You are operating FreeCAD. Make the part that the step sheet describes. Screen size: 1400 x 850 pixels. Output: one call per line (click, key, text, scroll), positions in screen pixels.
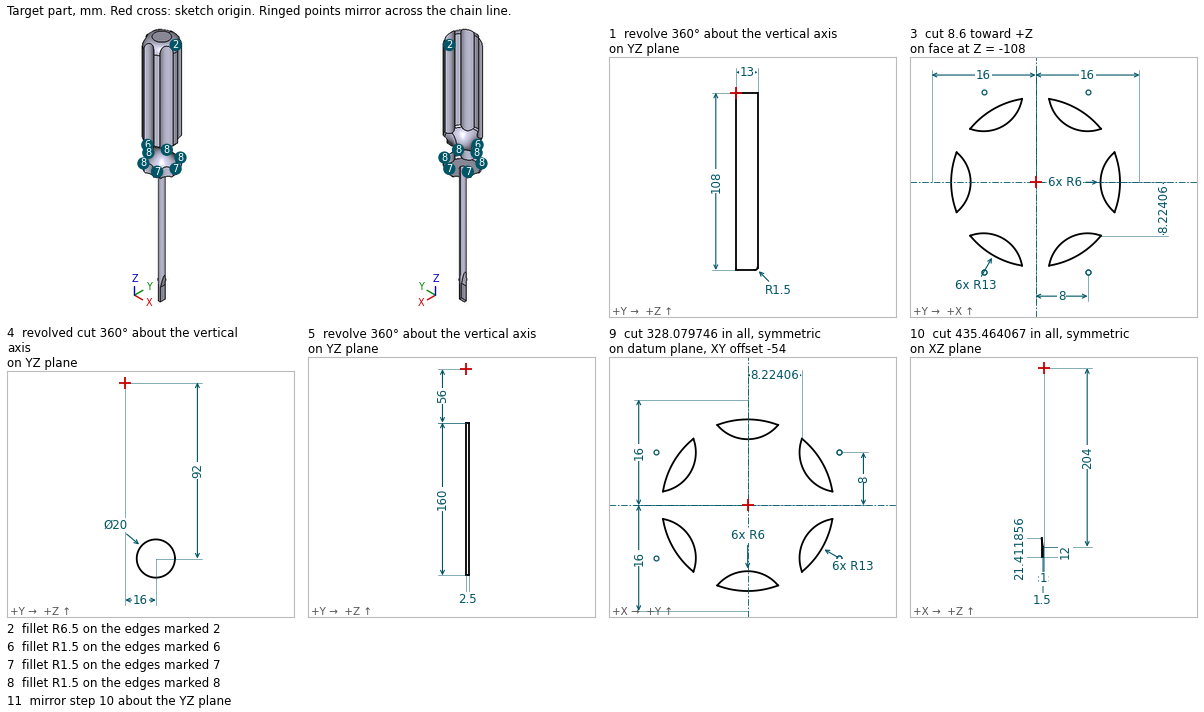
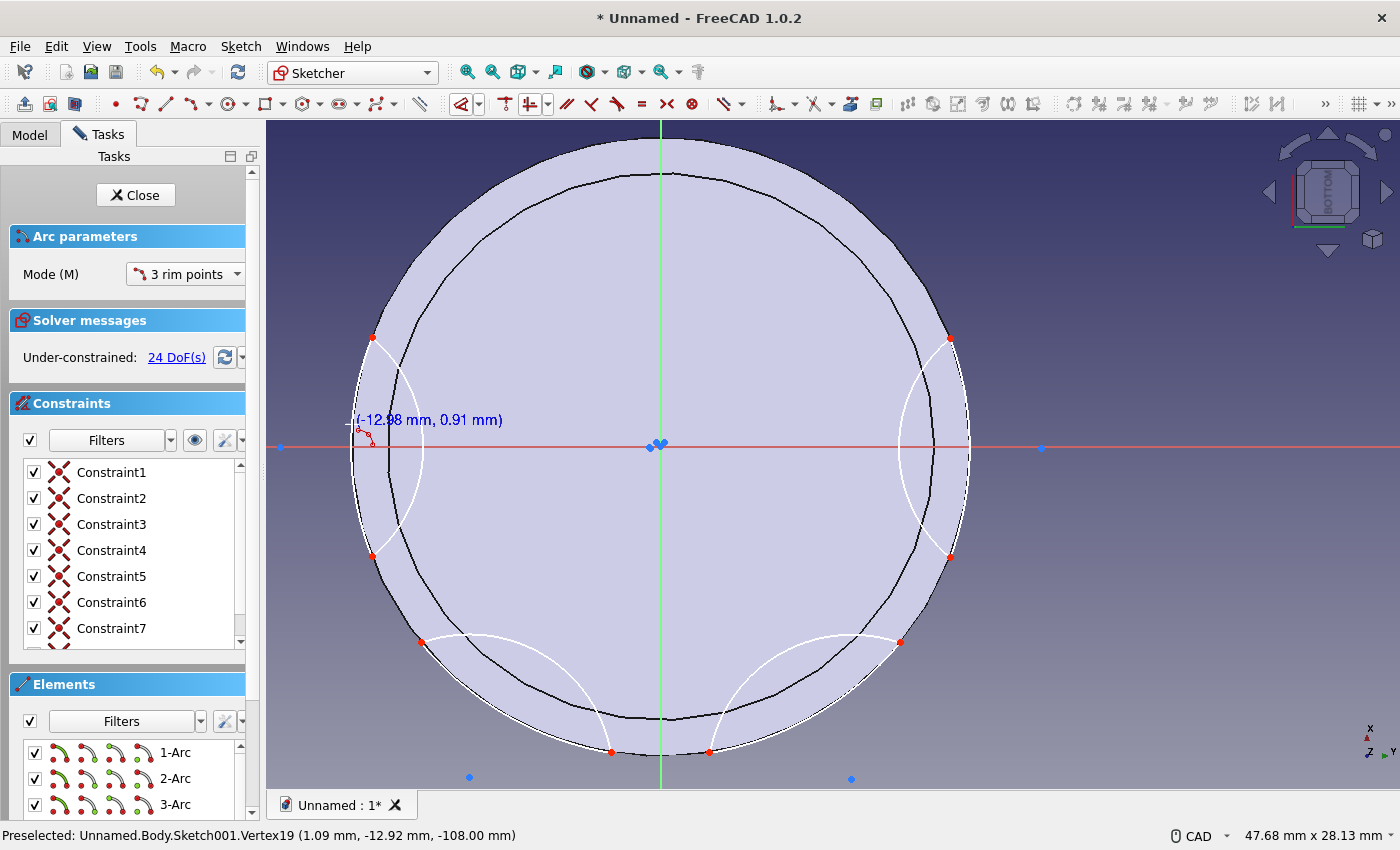
scroll(975, 471, down, 2)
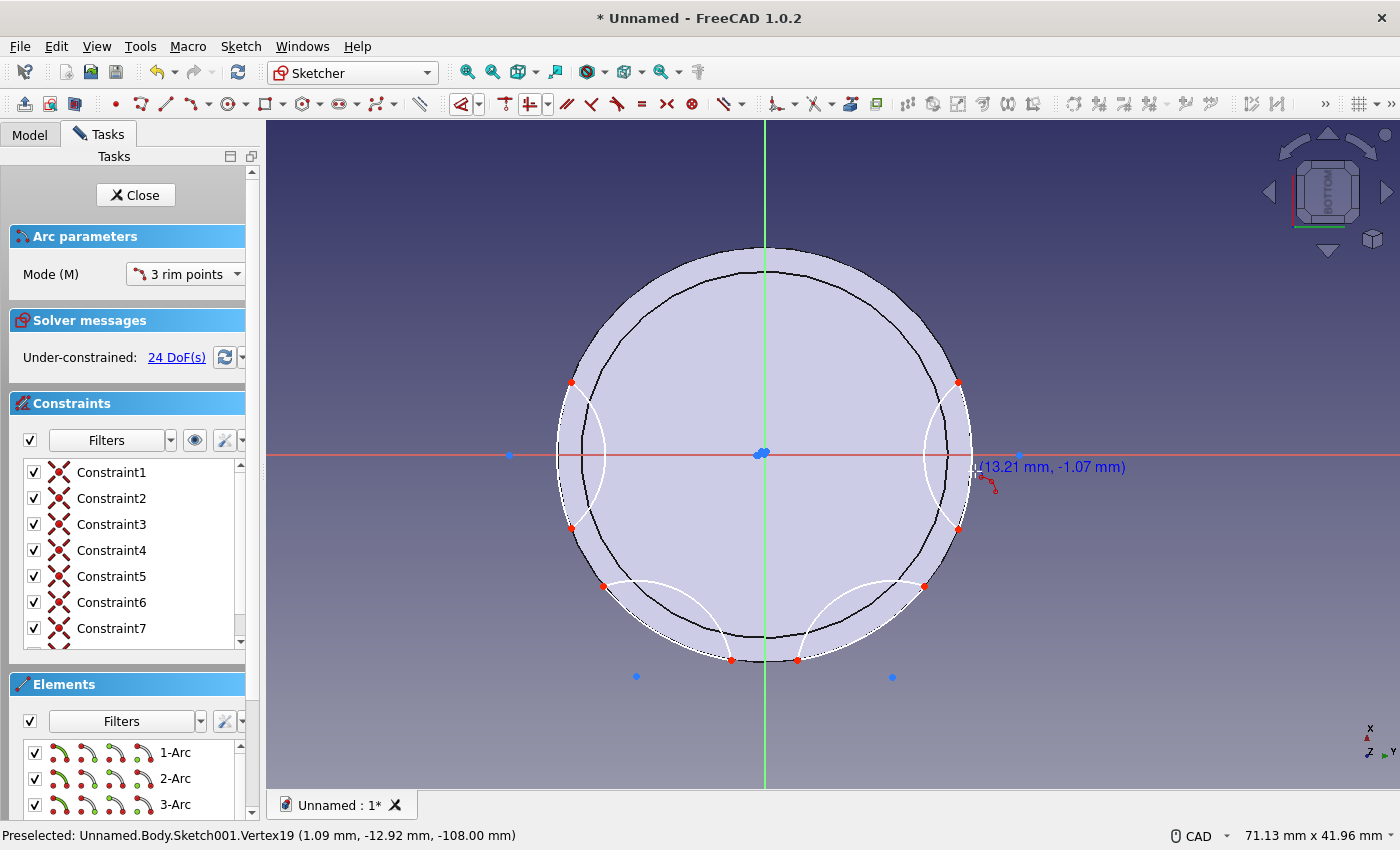
click(731, 250)
click(604, 324)
click(661, 275)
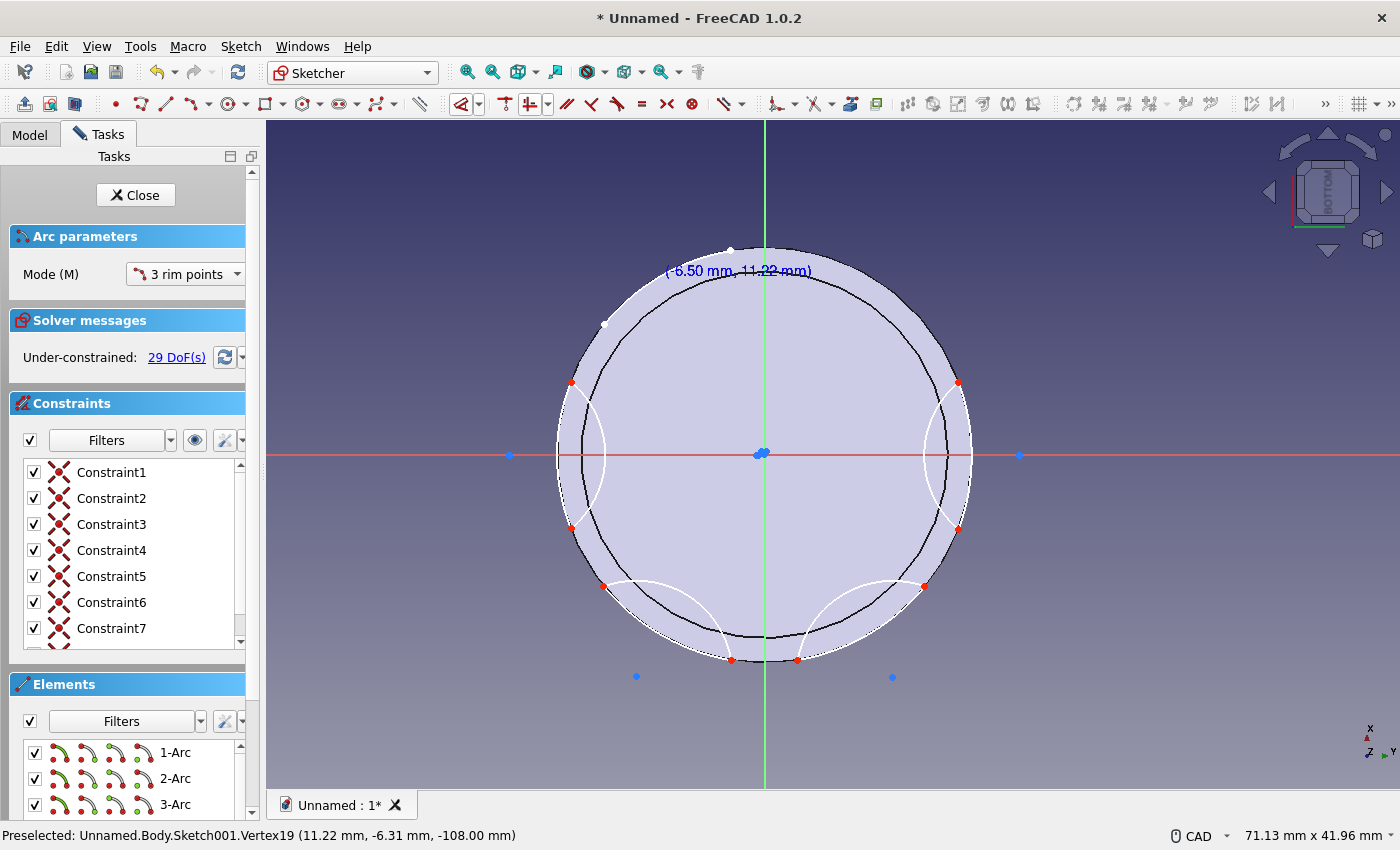
click(604, 325)
click(731, 251)
click(685, 317)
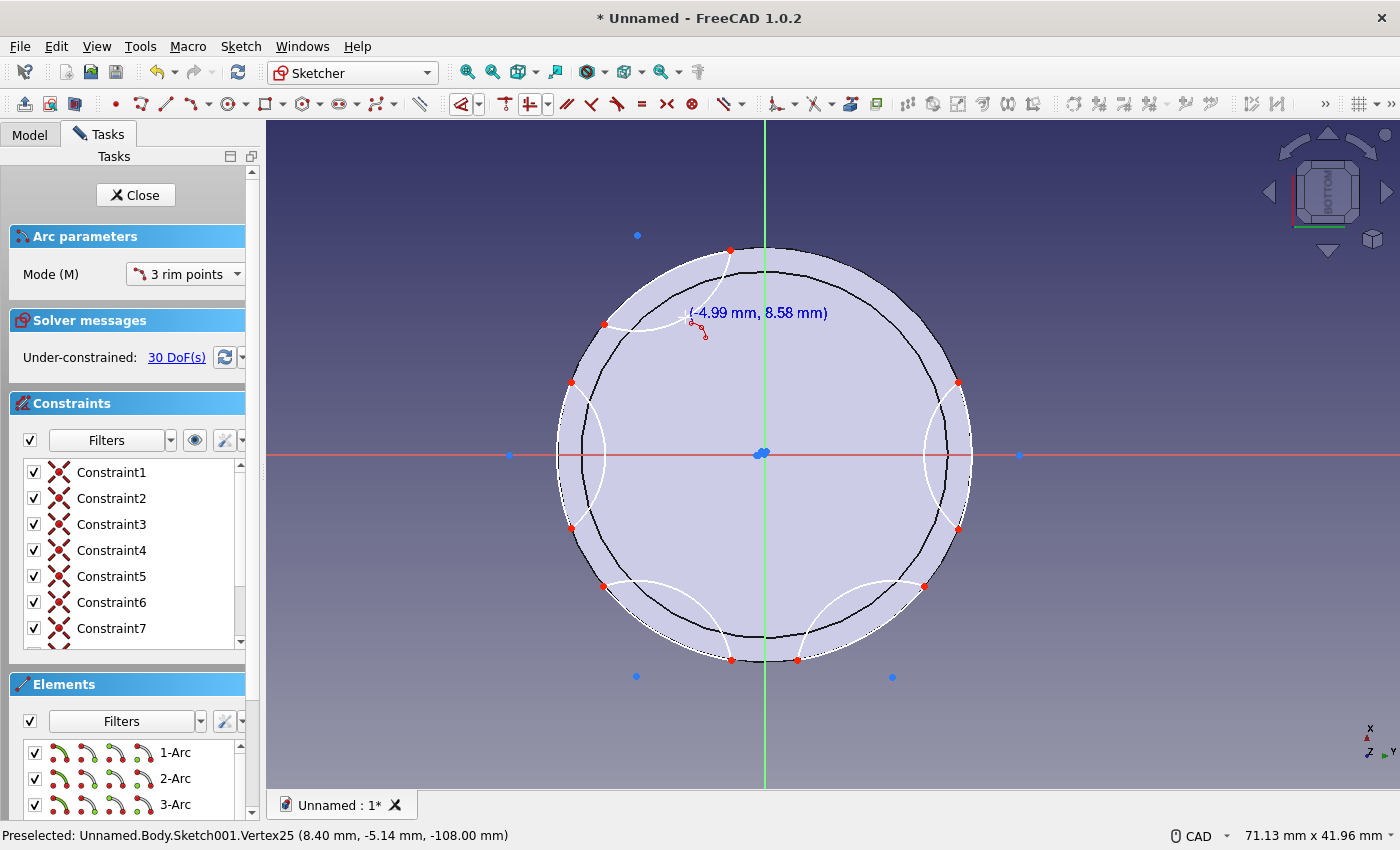
click(798, 250)
click(925, 324)
click(844, 317)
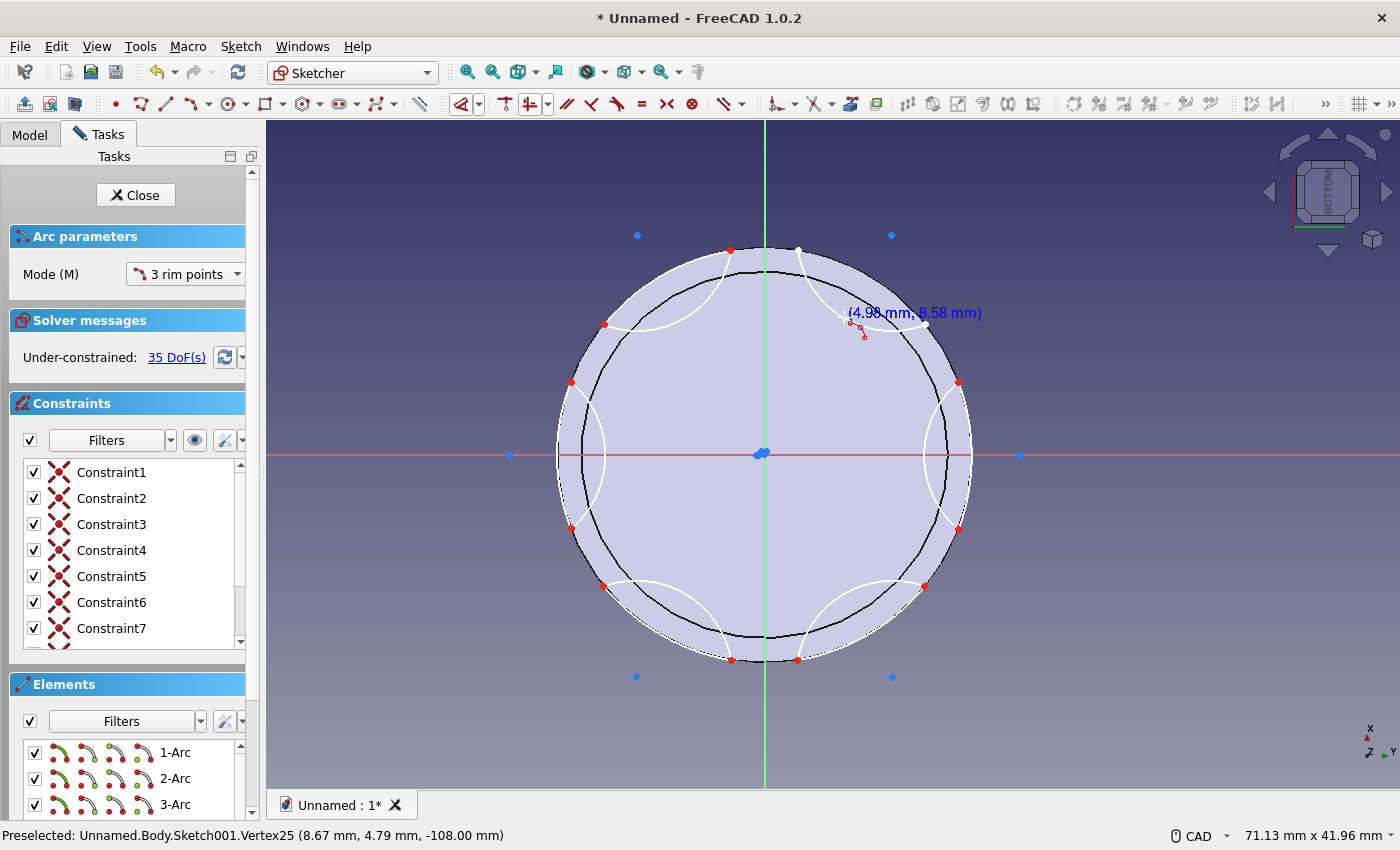
click(925, 325)
click(798, 251)
click(868, 275)
key(Escape)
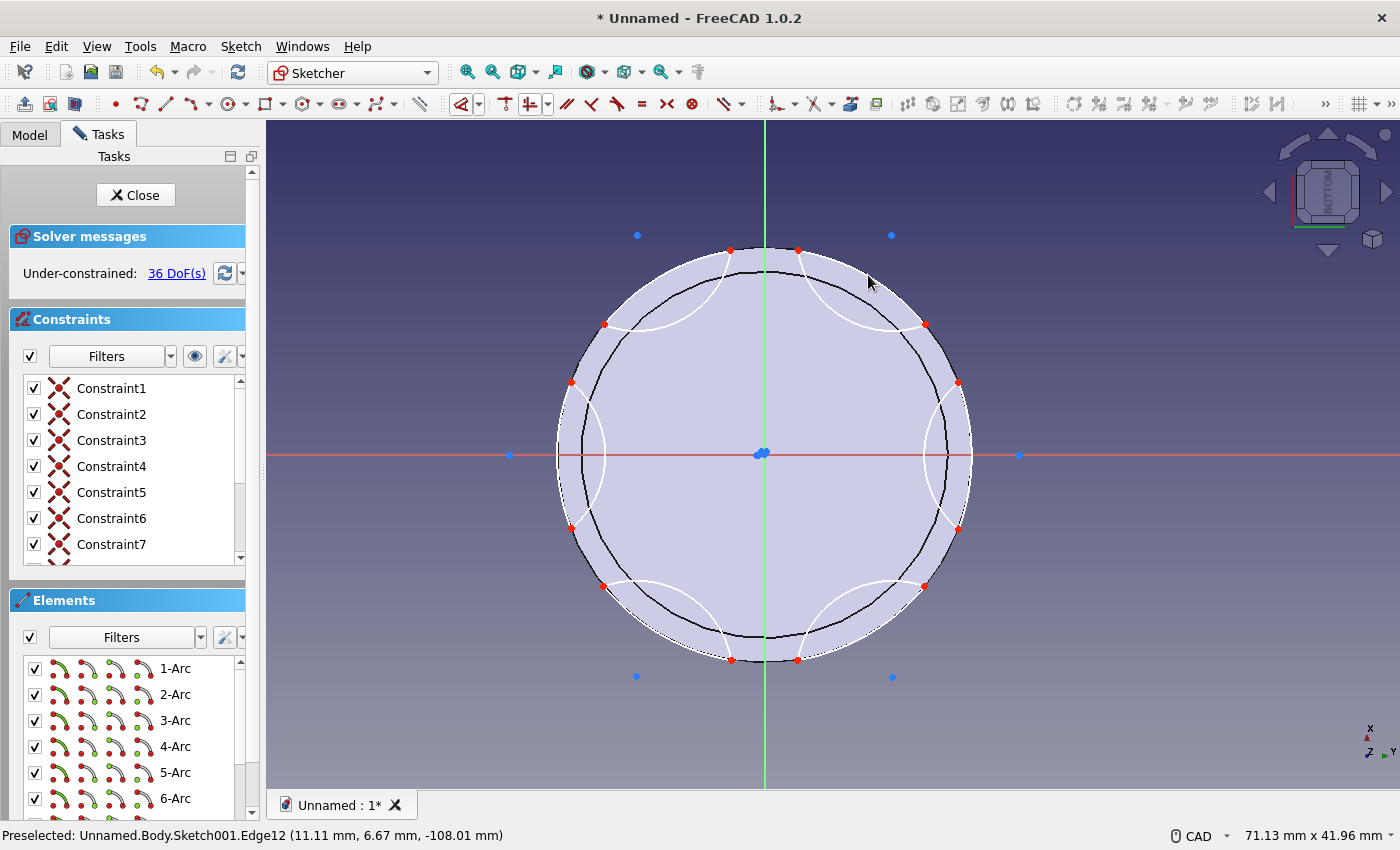
click(970, 486)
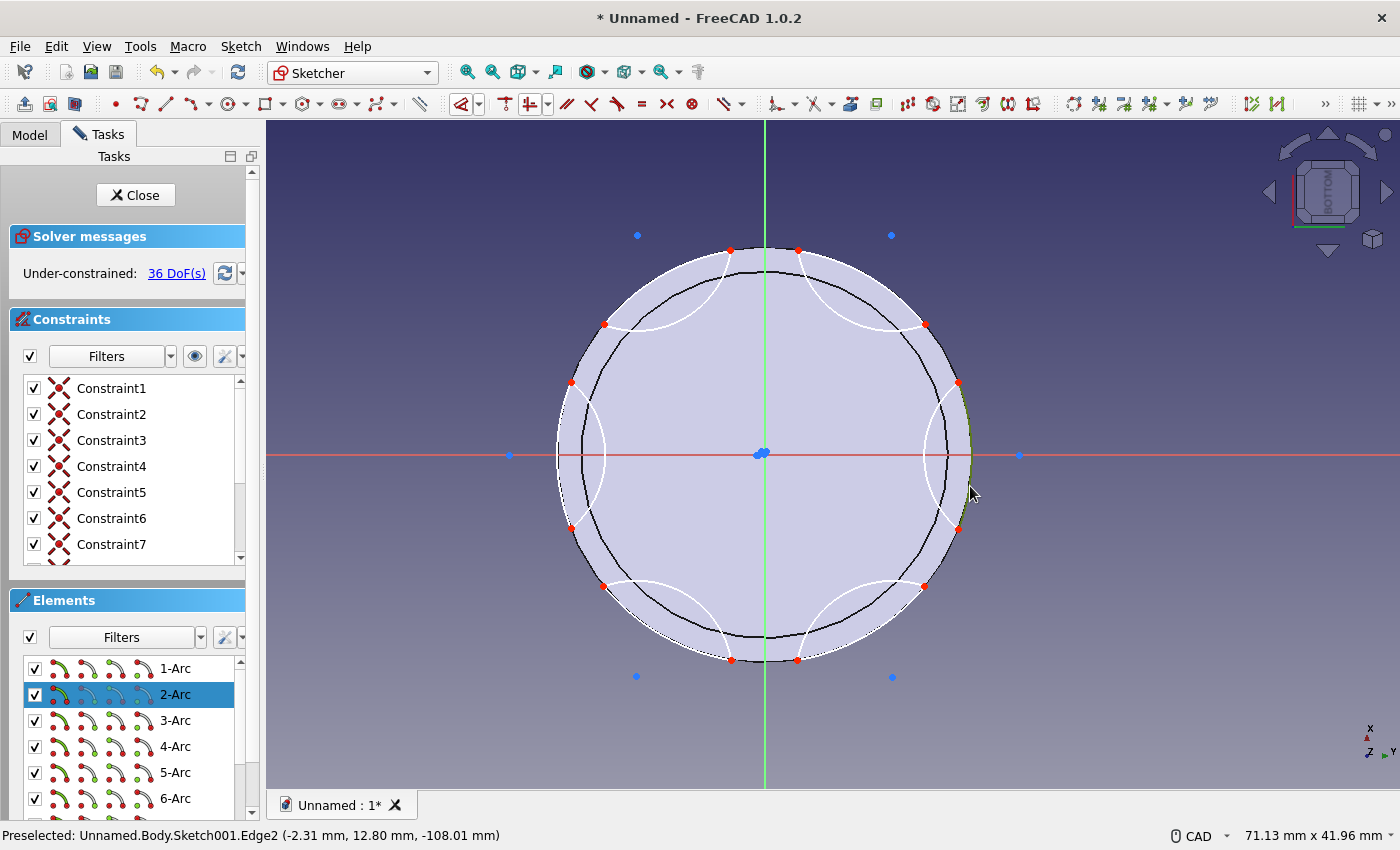
click(841, 648)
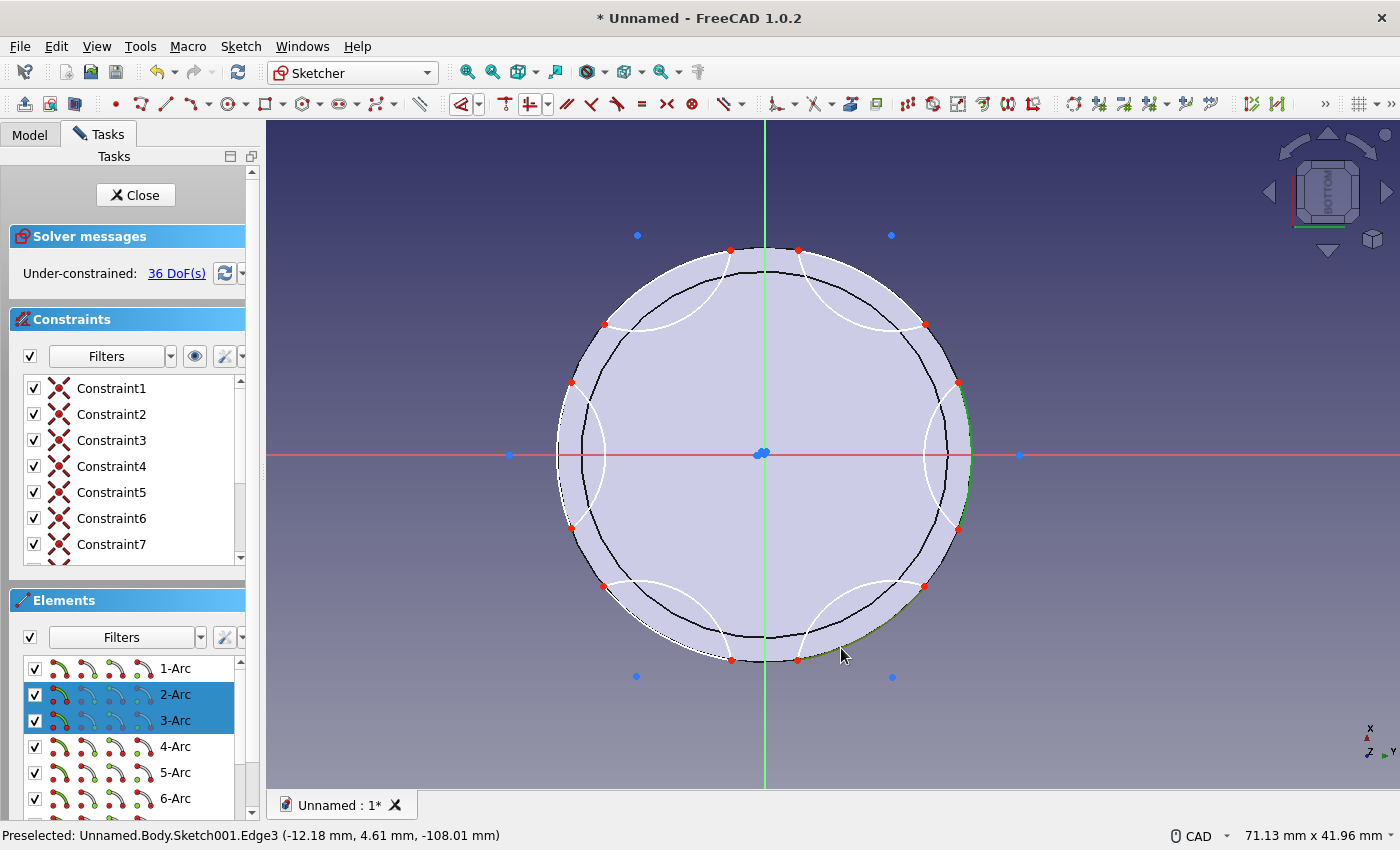
key(c)